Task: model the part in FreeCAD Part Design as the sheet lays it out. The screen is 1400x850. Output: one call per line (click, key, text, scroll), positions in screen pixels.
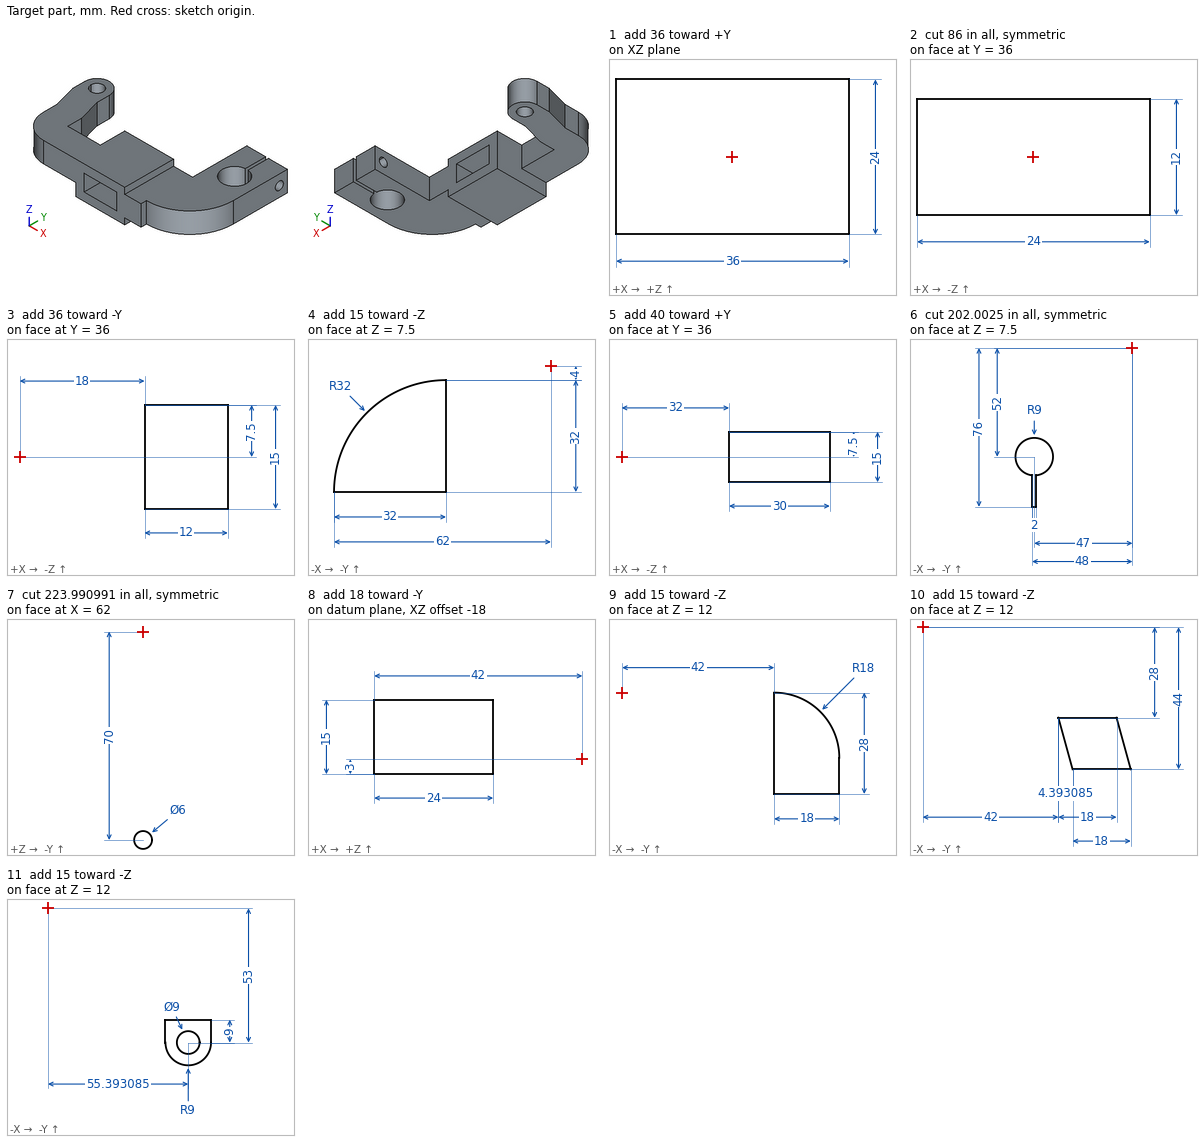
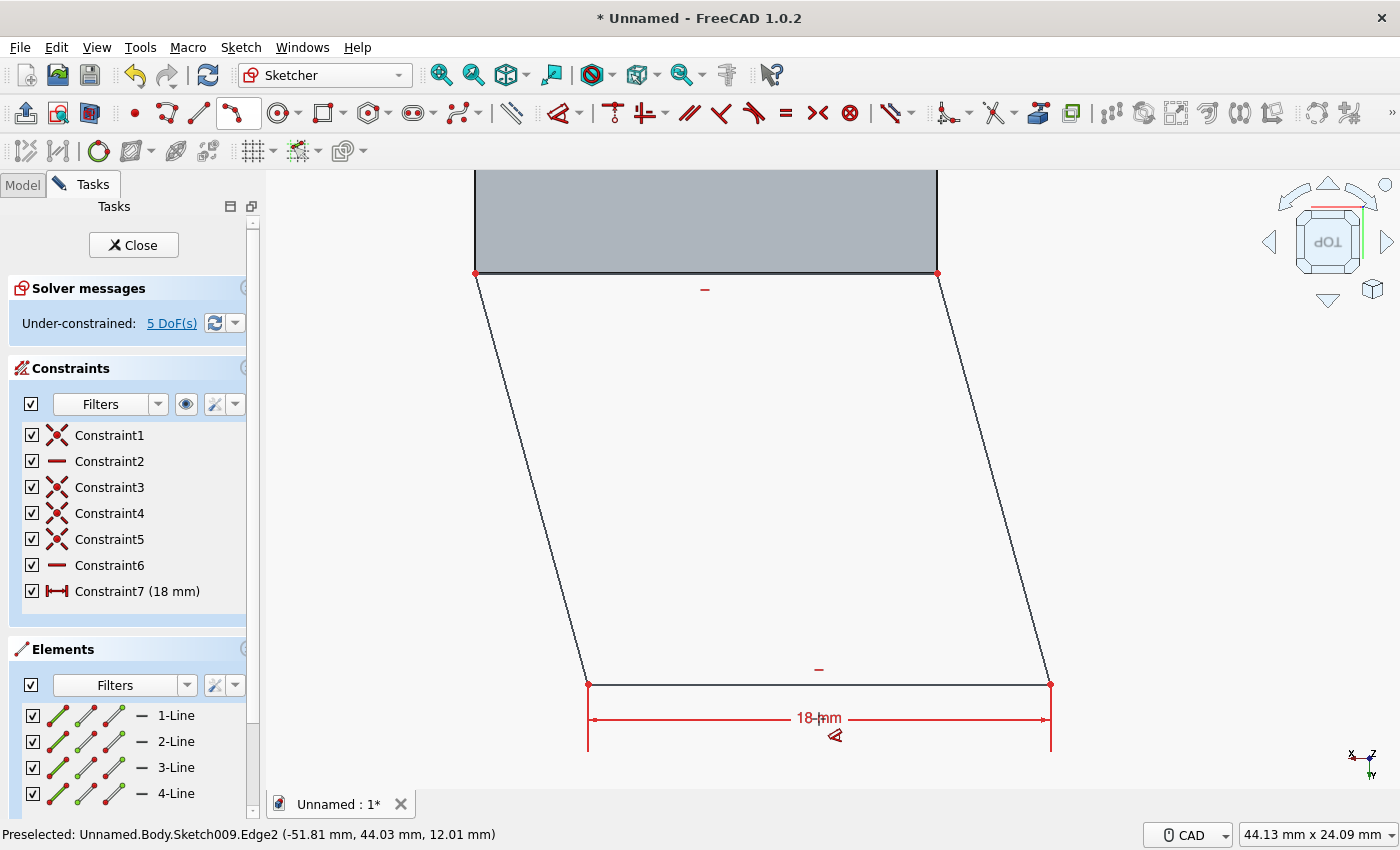
click(798, 274)
click(706, 240)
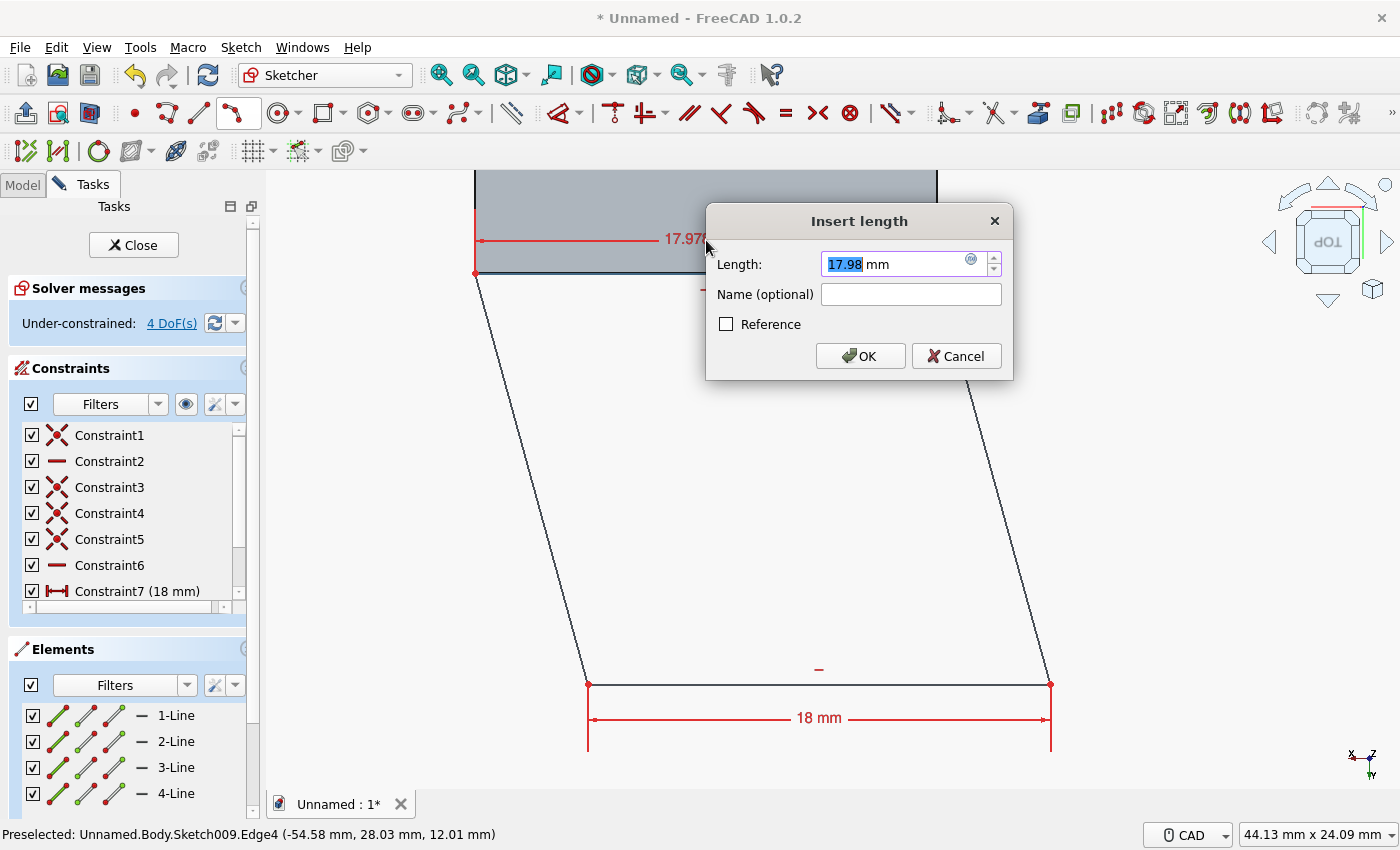
text(18)
key(Return)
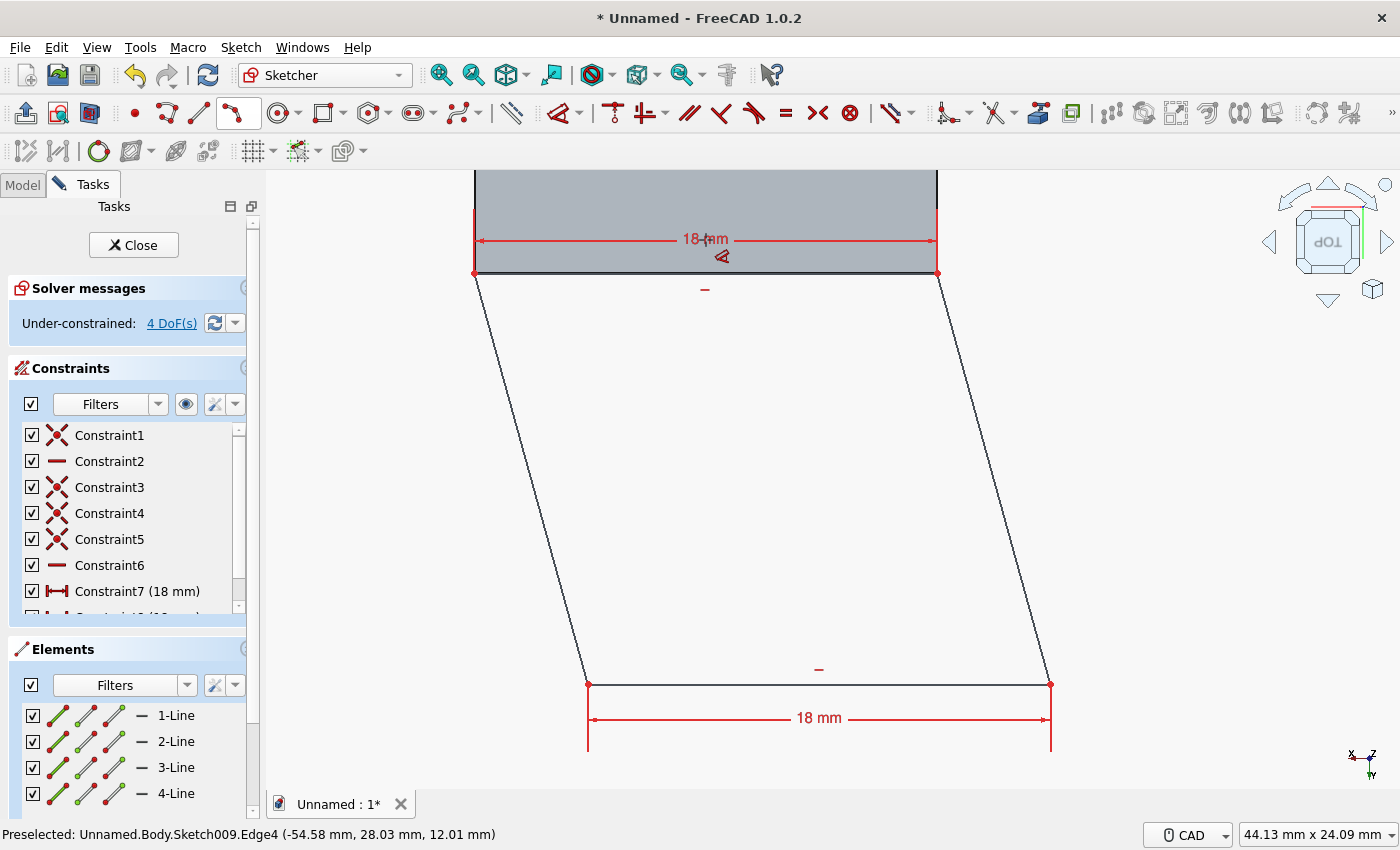
click(474, 274)
click(384, 308)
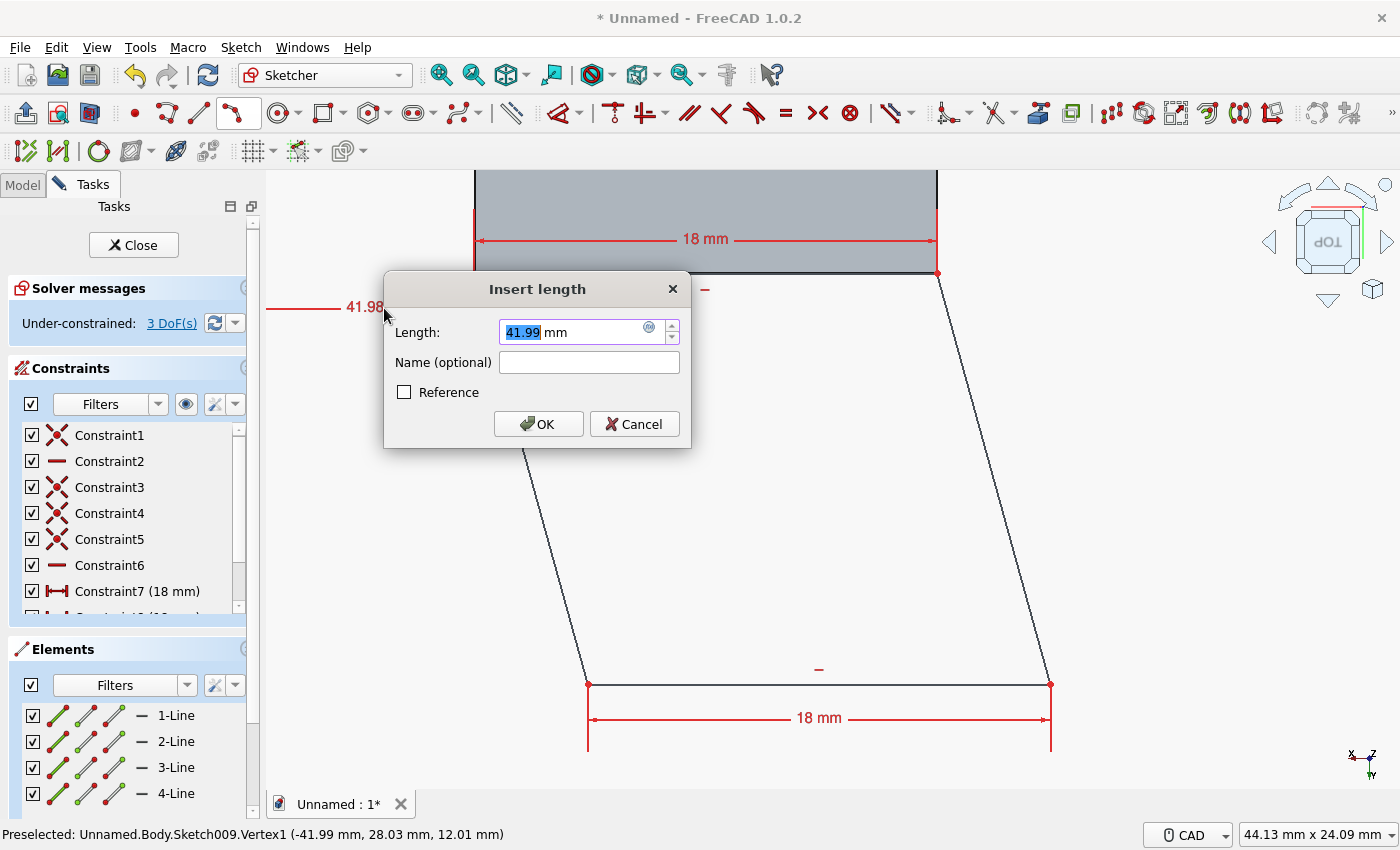
text(42)
key(Return)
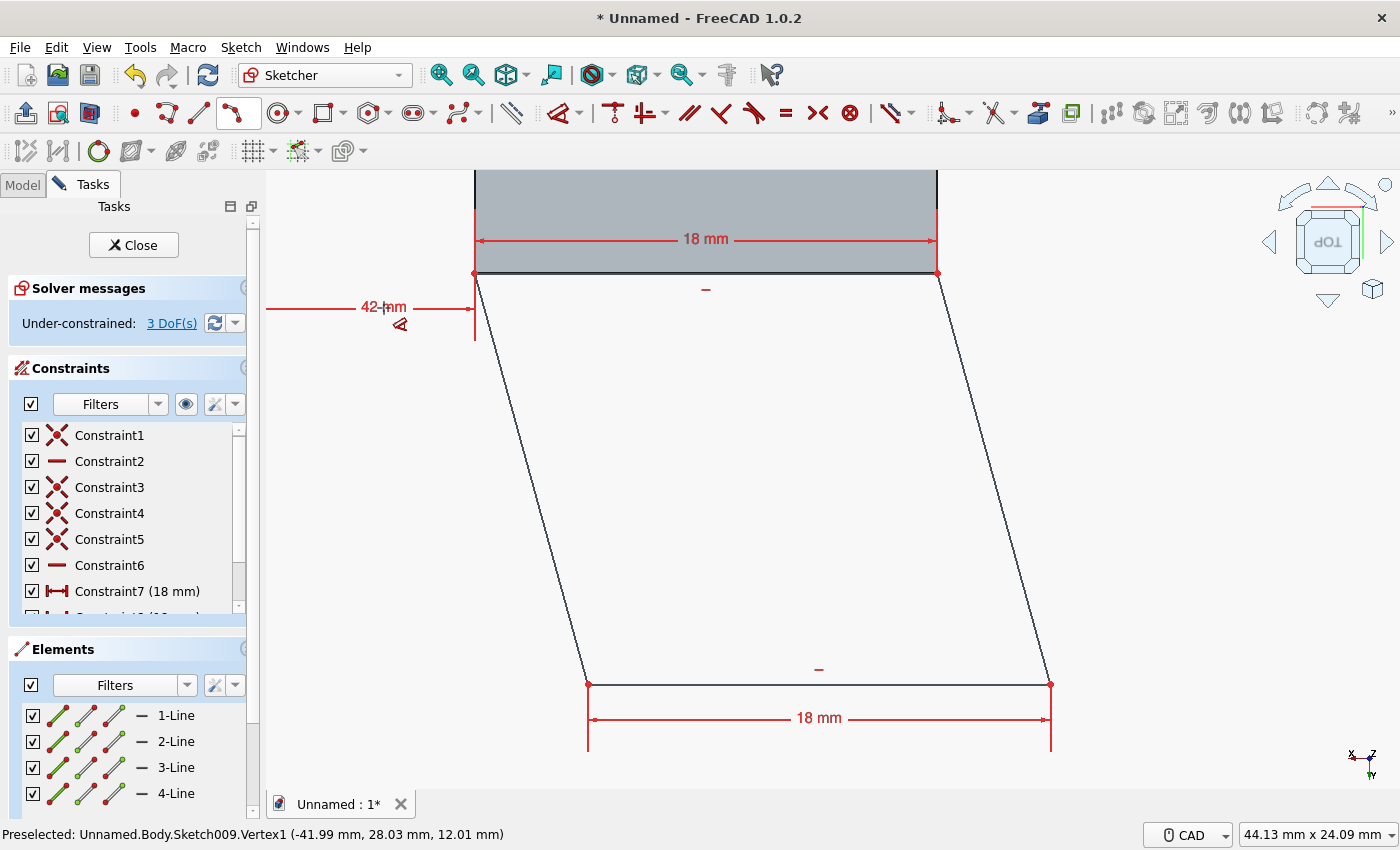
click(475, 274)
click(509, 236)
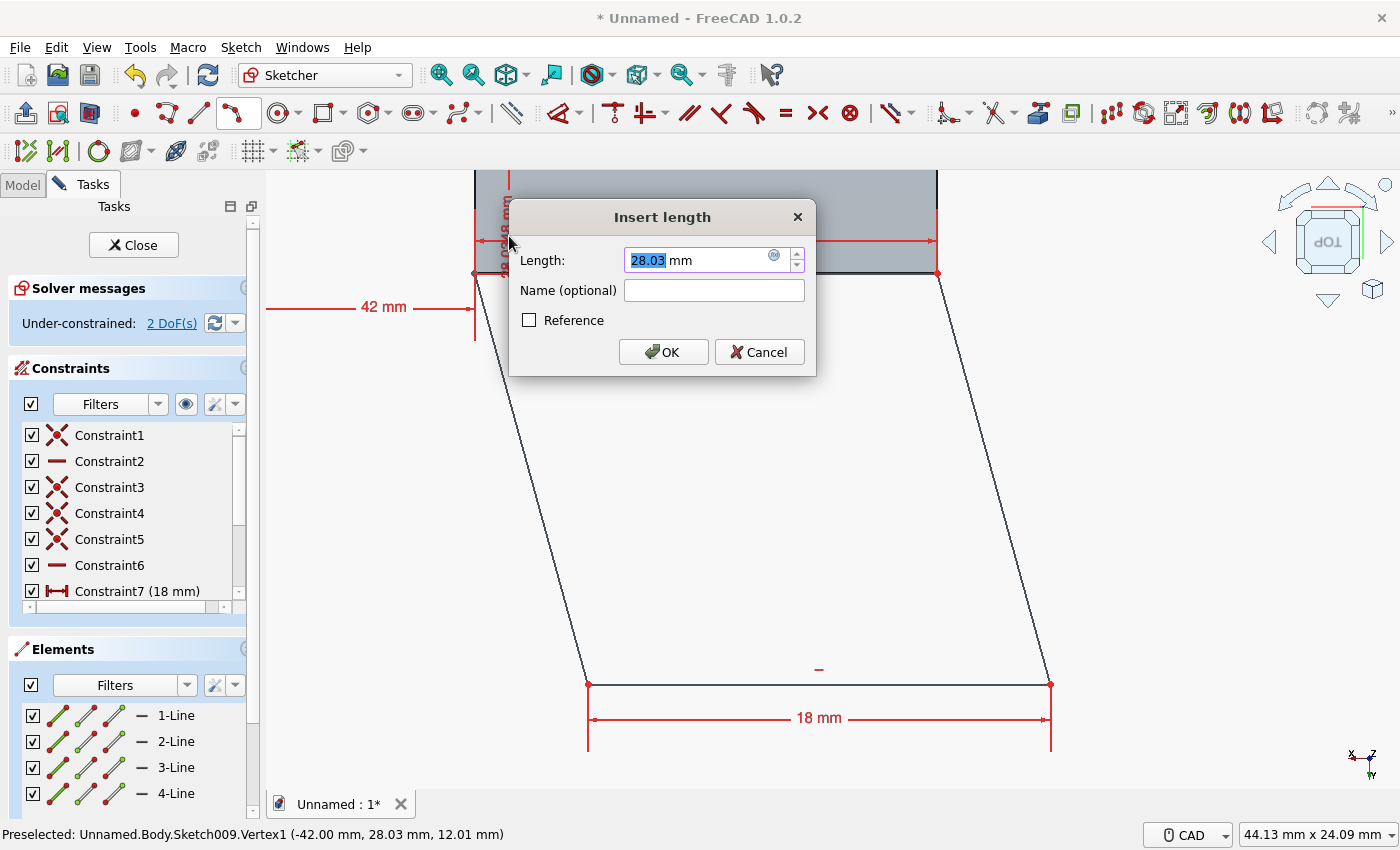
text(28)
key(Return)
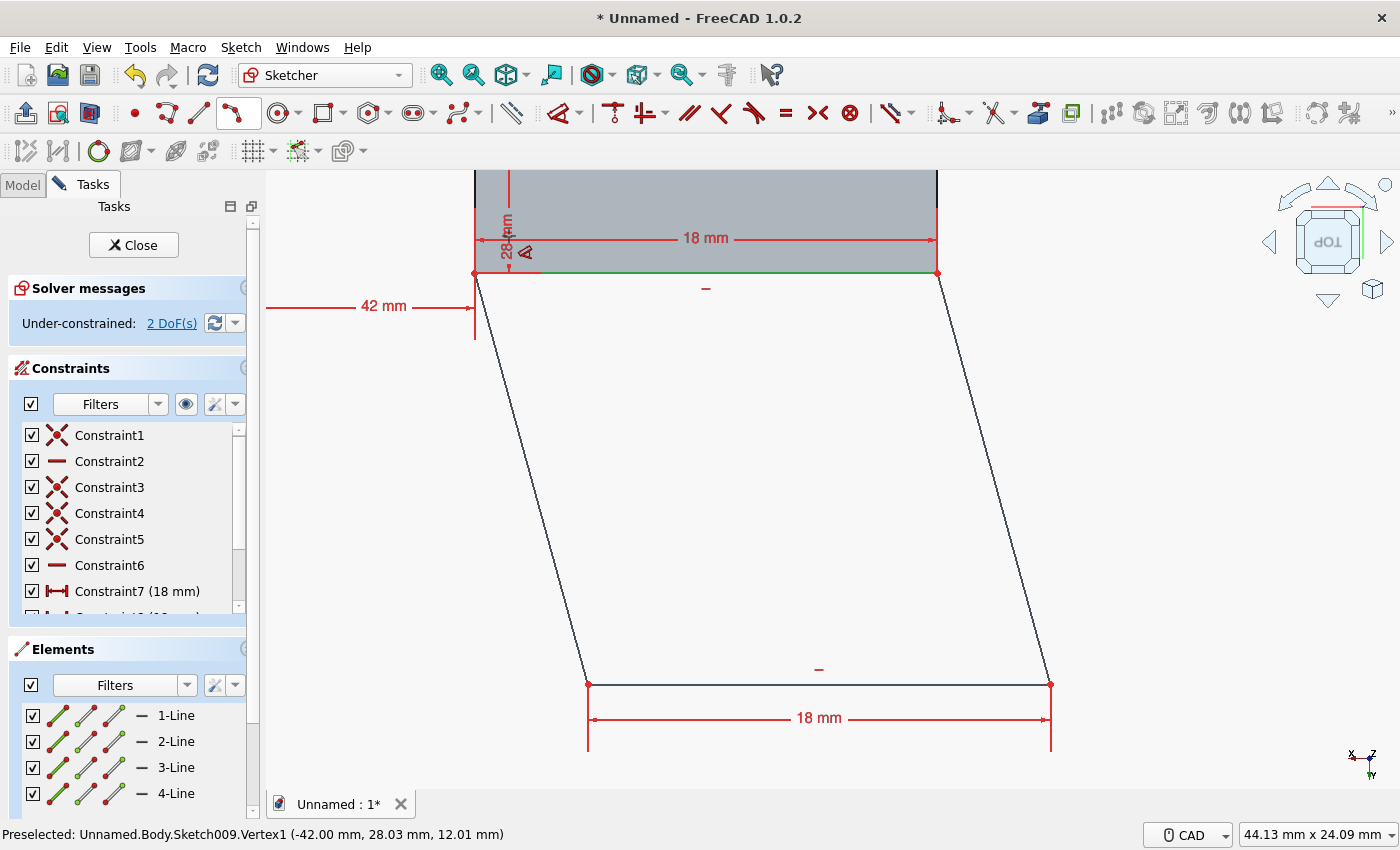
click(588, 685)
click(622, 442)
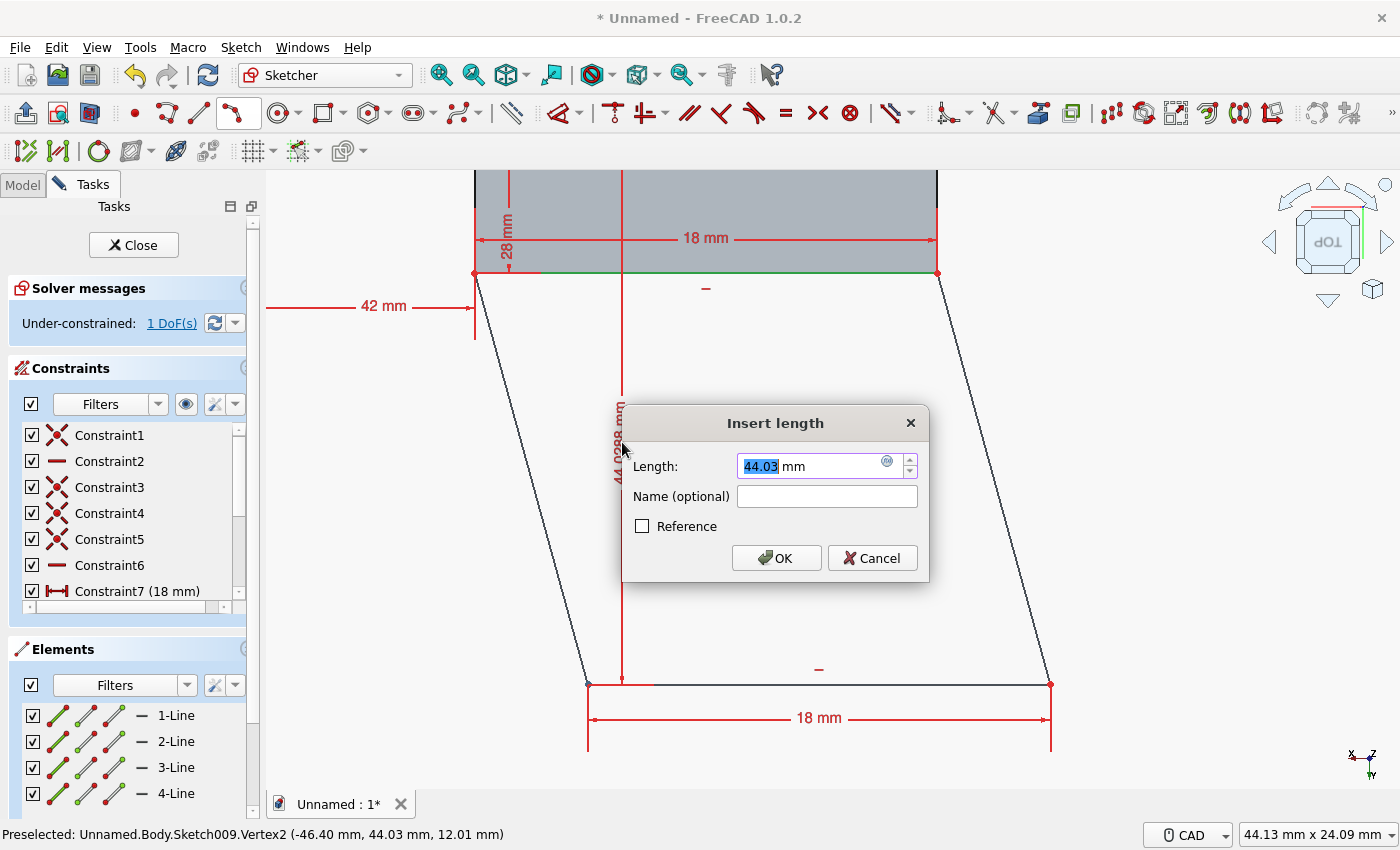
text(44)
key(Return)